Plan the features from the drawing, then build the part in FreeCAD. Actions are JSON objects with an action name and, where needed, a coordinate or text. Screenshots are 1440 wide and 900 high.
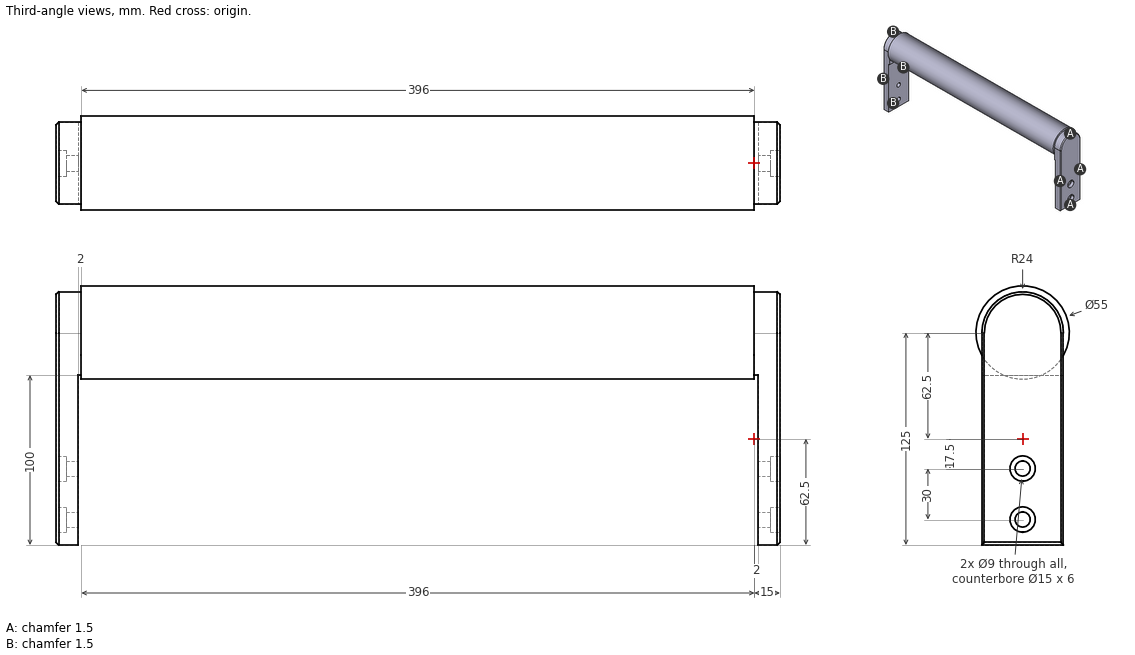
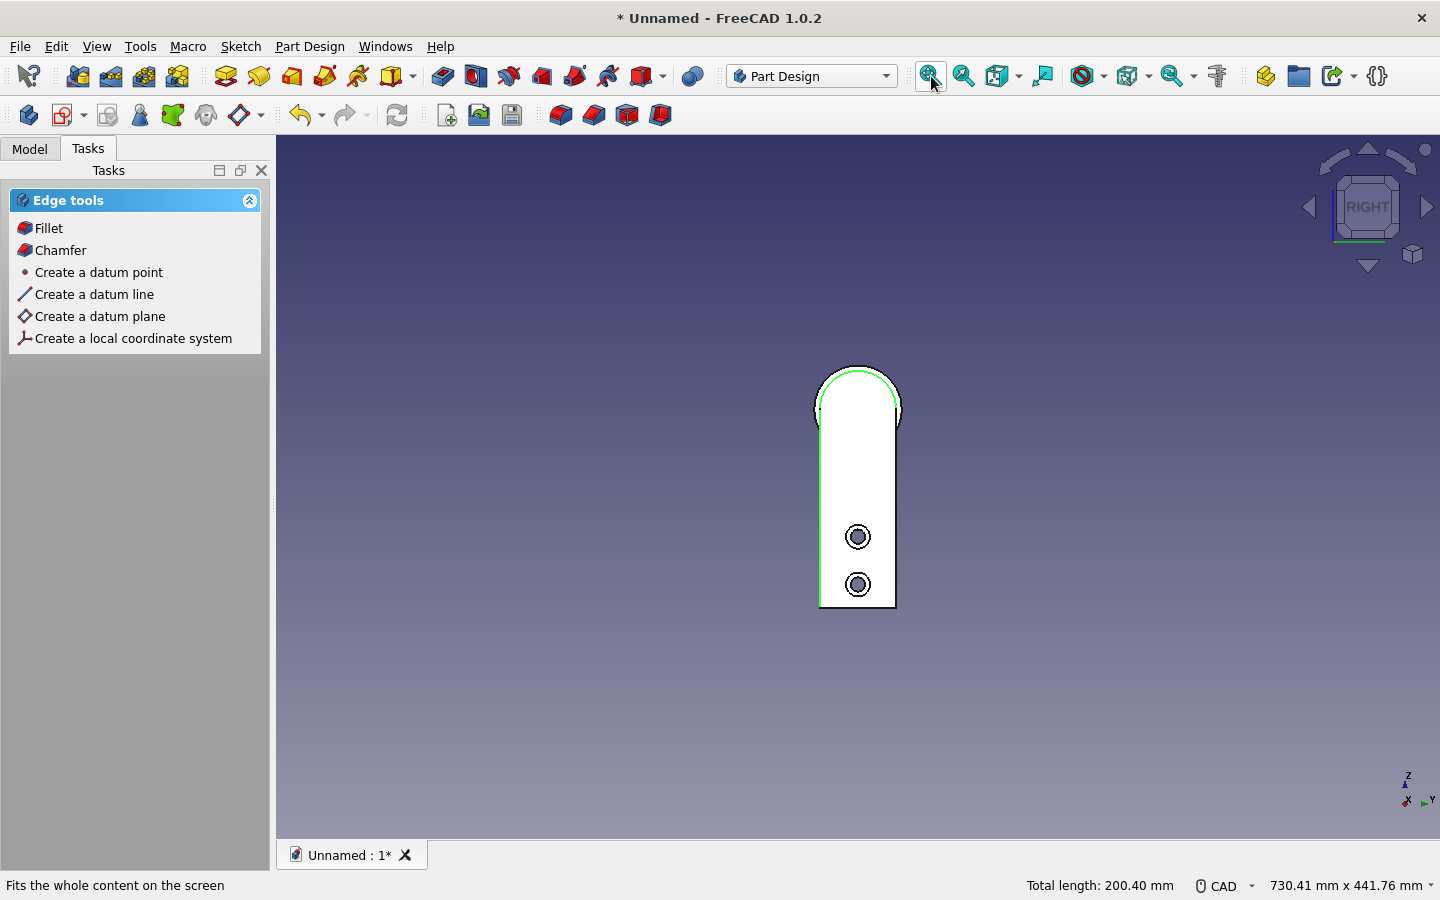
{"action": "left_click", "coordinate": [858, 607], "text": "ctrl"}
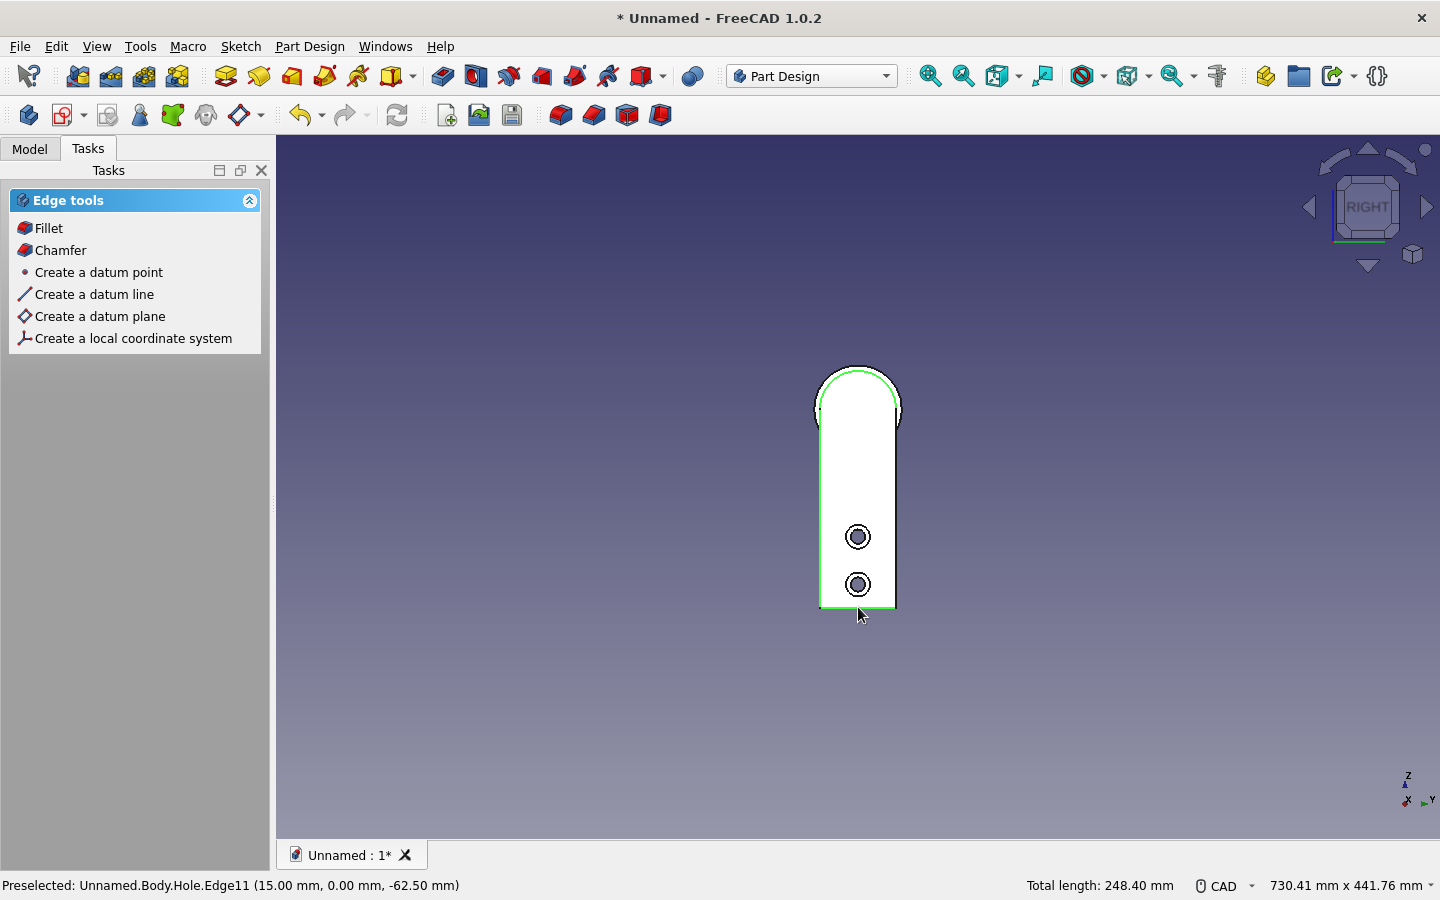
{"action": "left_click", "coordinate": [896, 508], "text": "ctrl"}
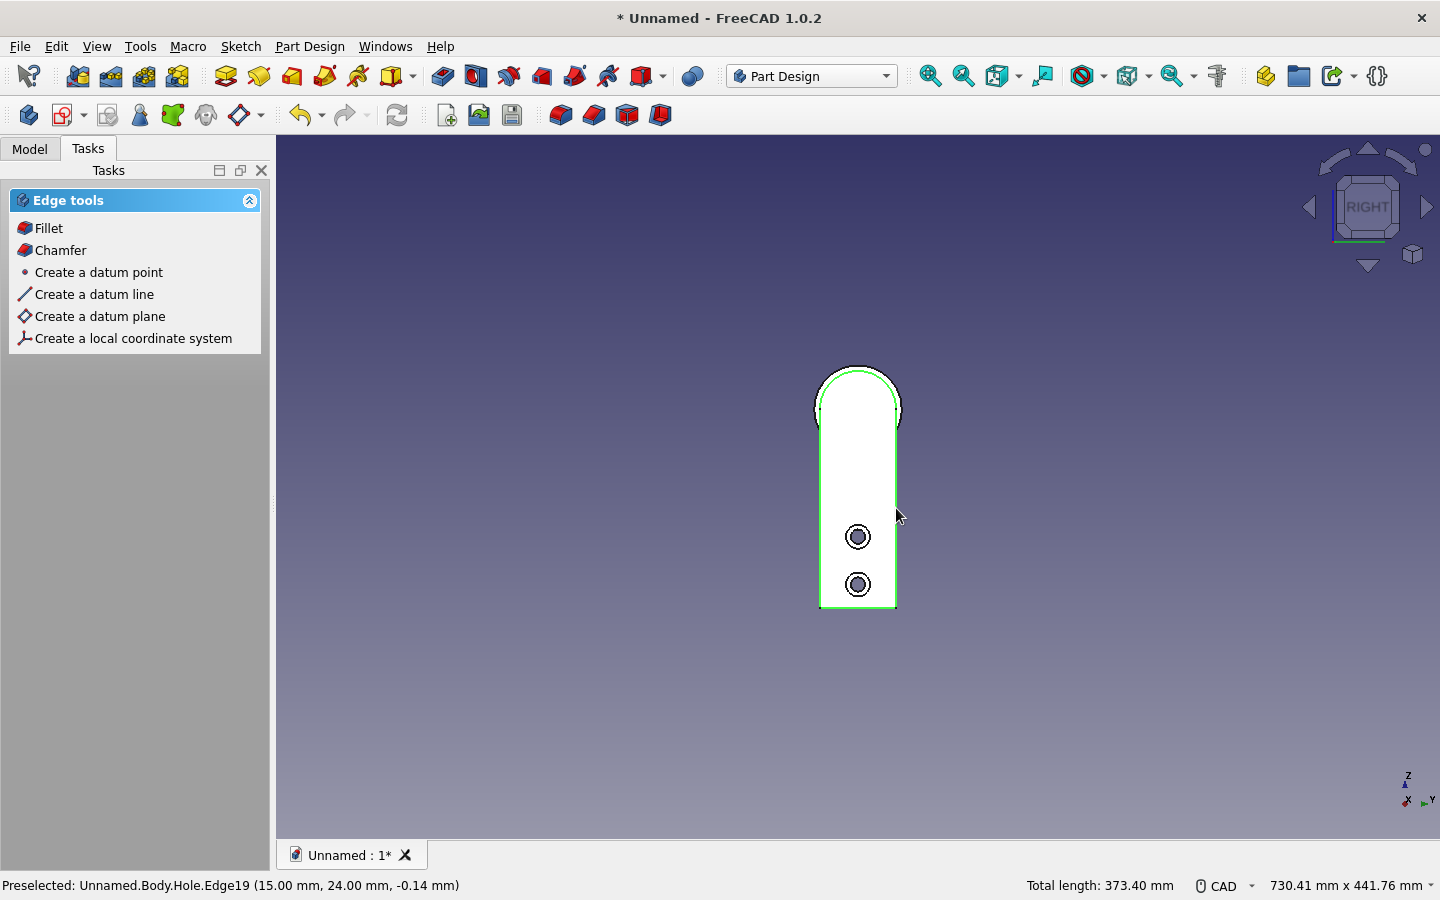
{"action": "left_click", "coordinate": [594, 116]}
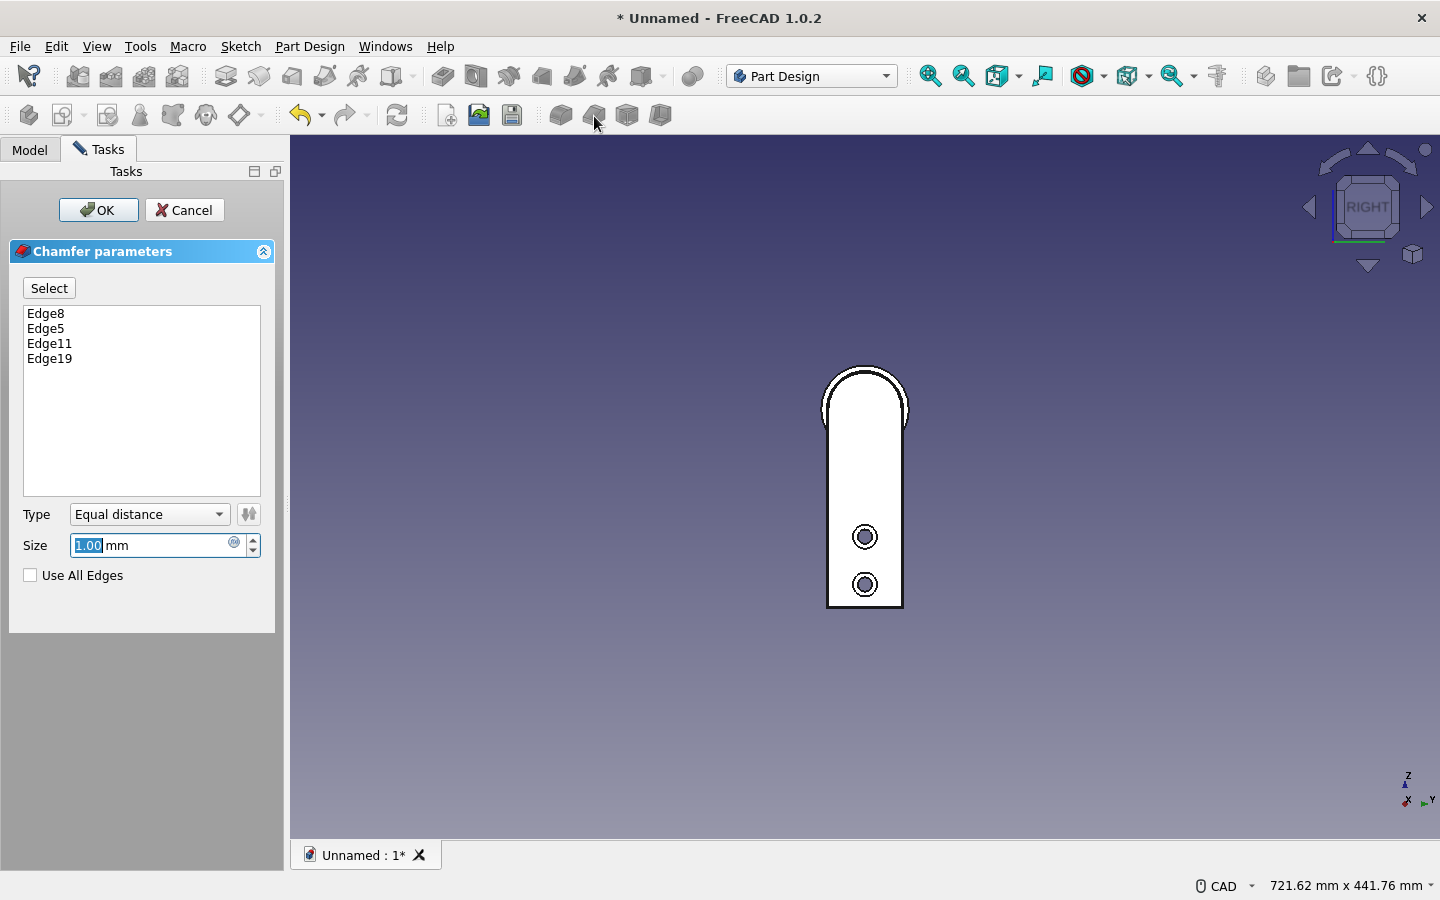
{"action": "type", "text": "1.5"}
{"action": "key", "text": "Tab"}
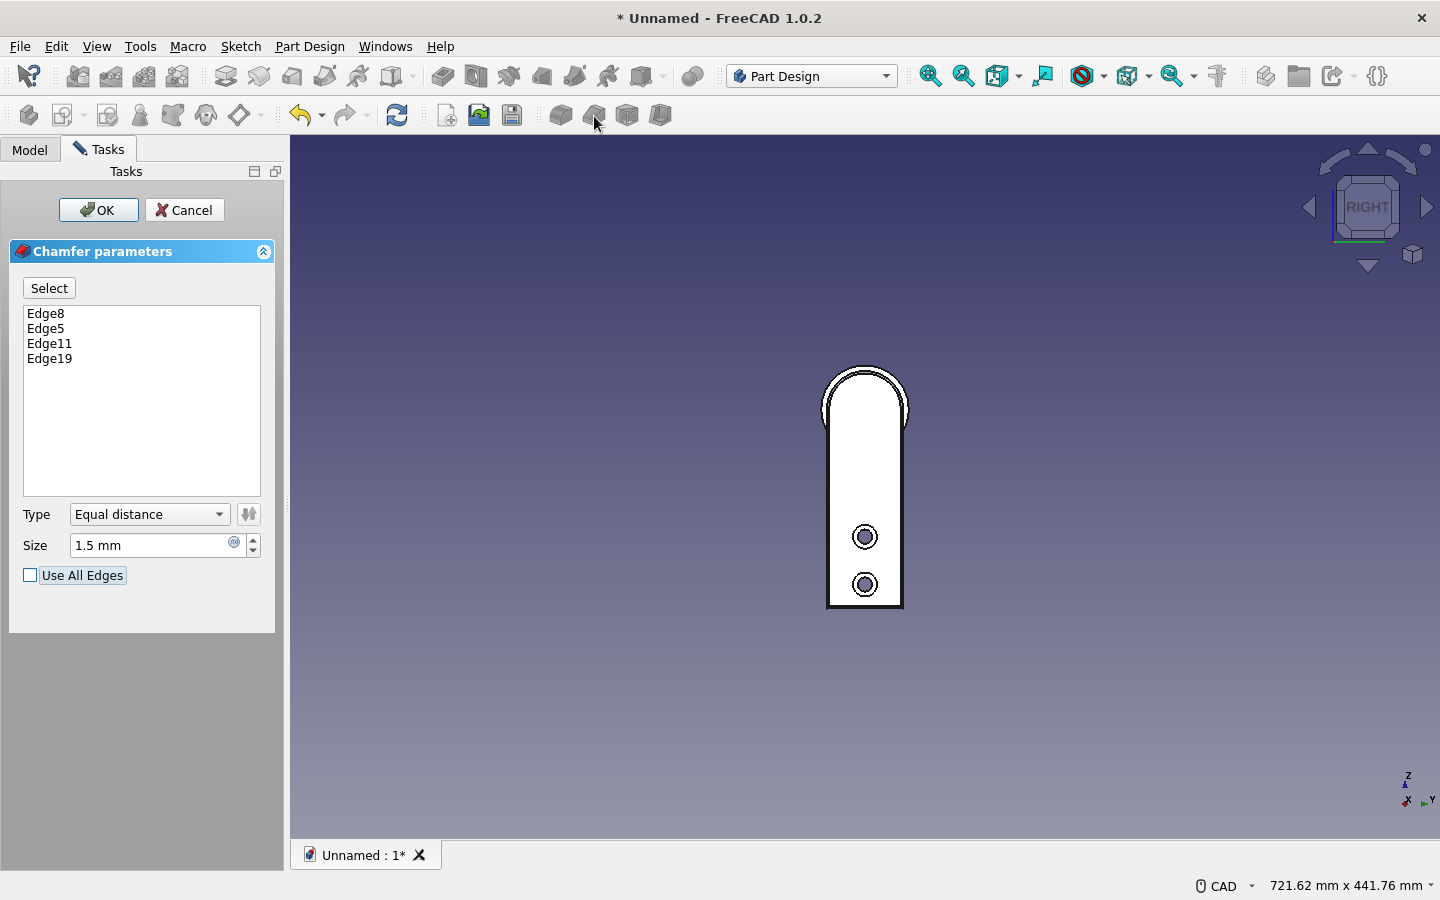
{"action": "left_click", "coordinate": [99, 210]}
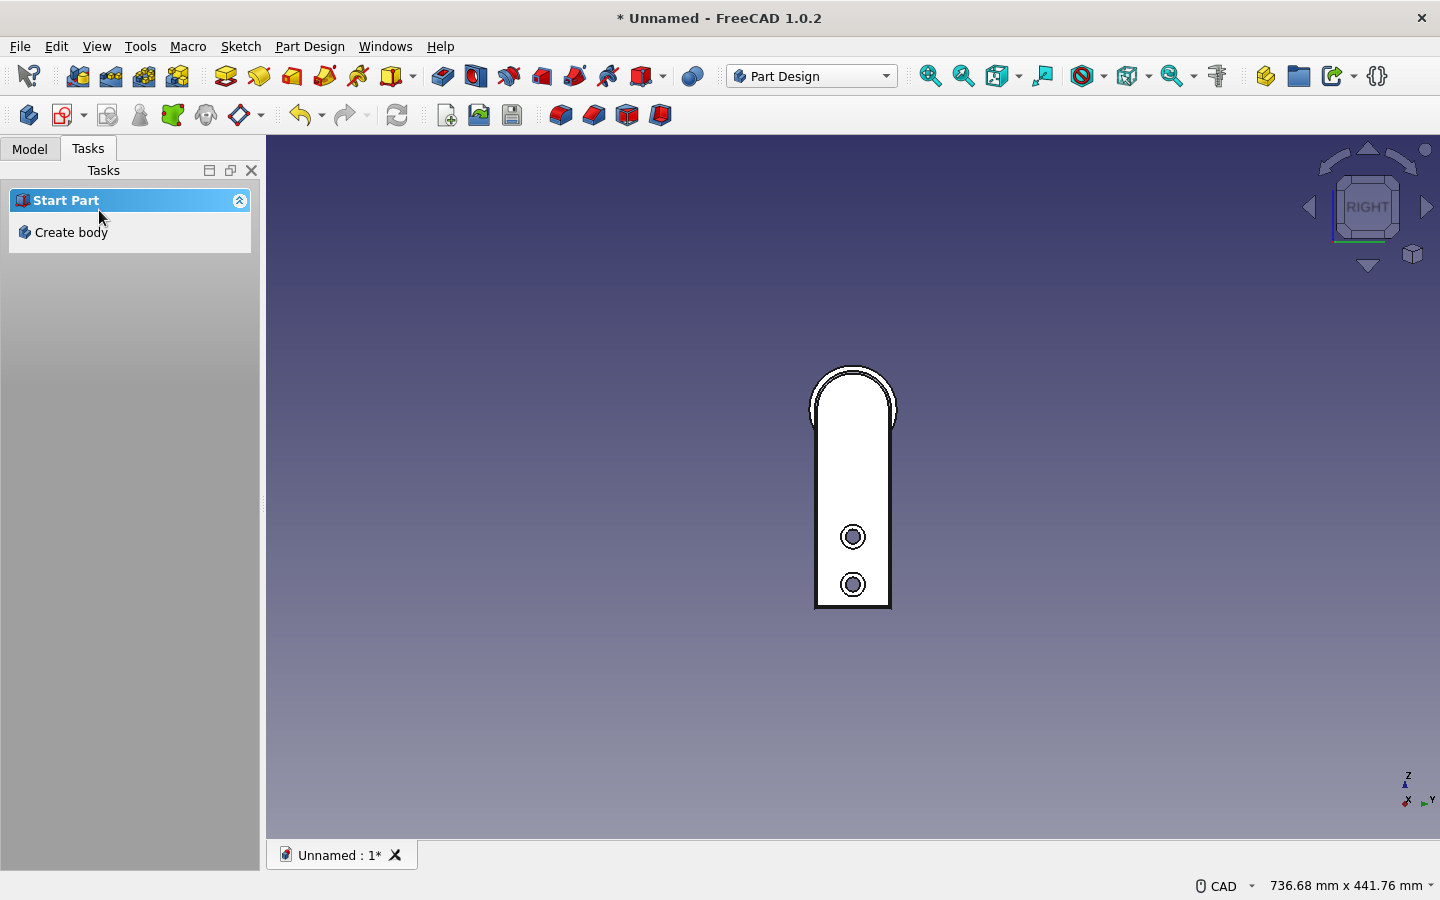
{"action": "left_click", "coordinate": [931, 76]}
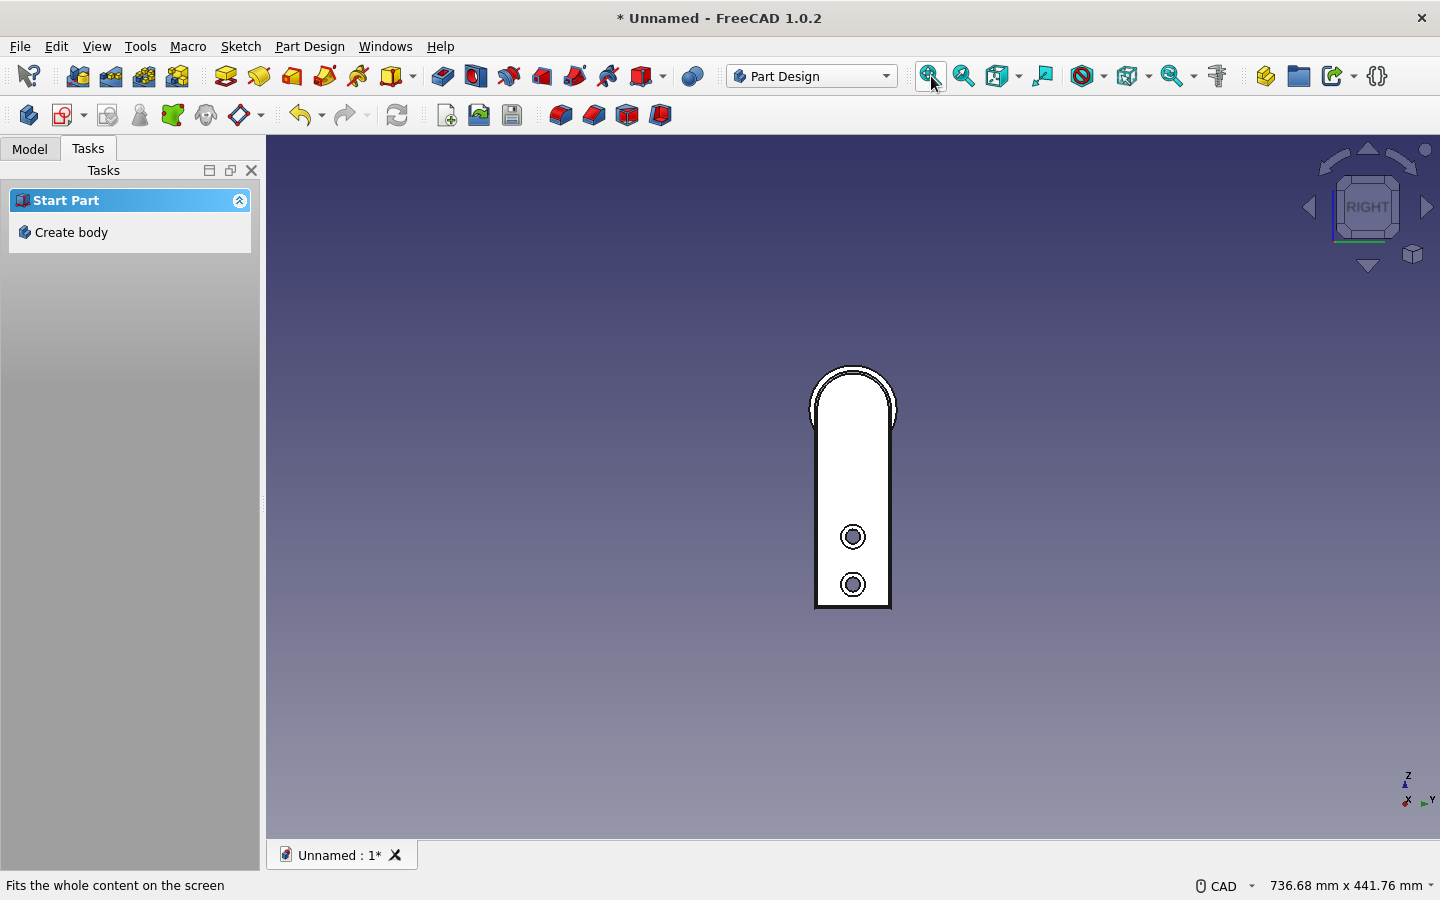
{"action": "left_click", "coordinate": [30, 148]}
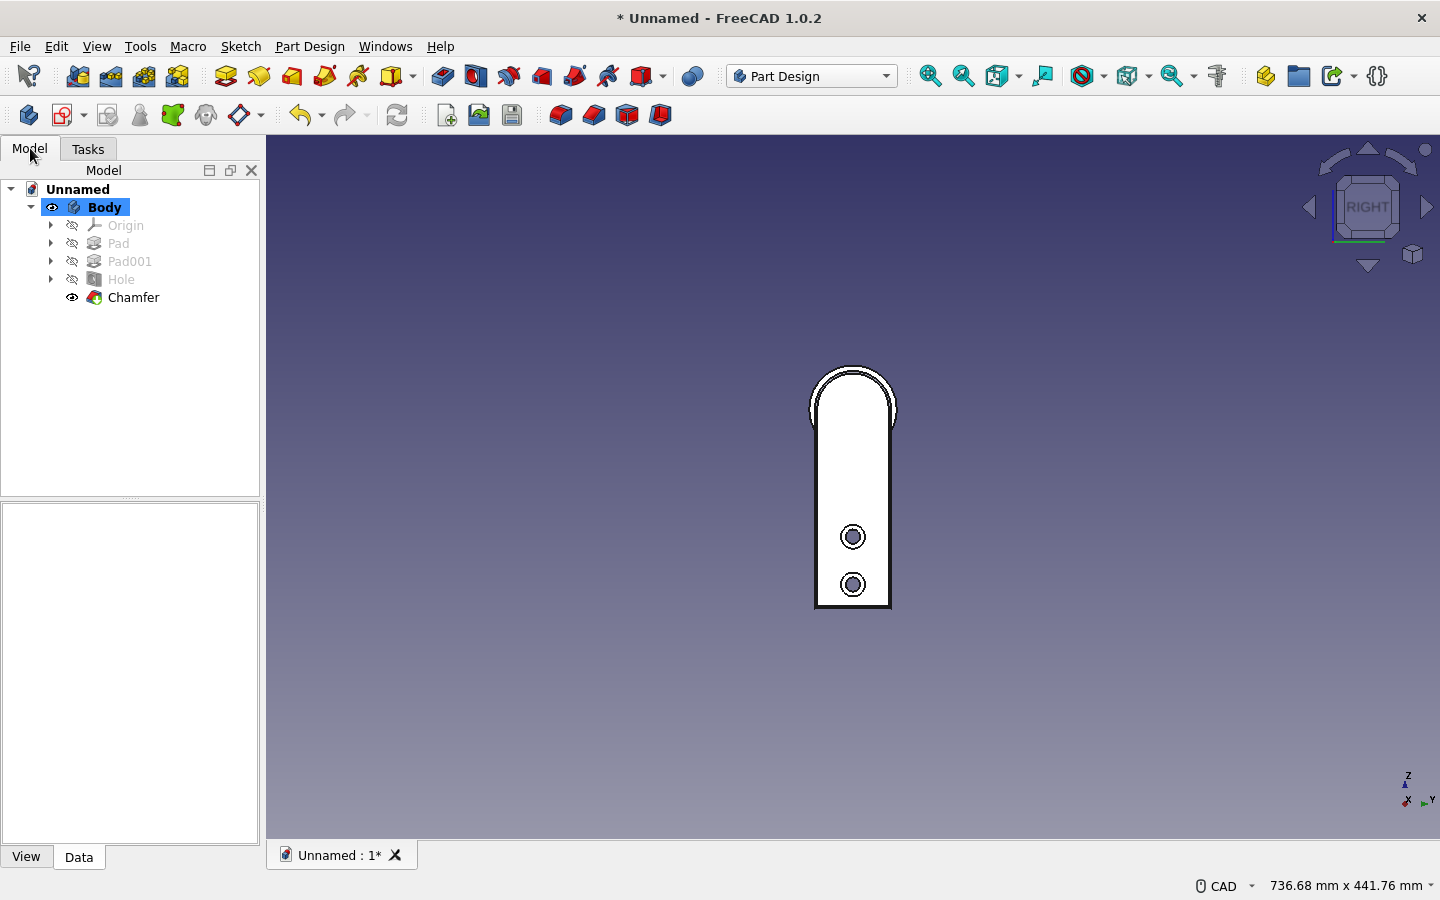
{"action": "left_click", "coordinate": [51, 225]}